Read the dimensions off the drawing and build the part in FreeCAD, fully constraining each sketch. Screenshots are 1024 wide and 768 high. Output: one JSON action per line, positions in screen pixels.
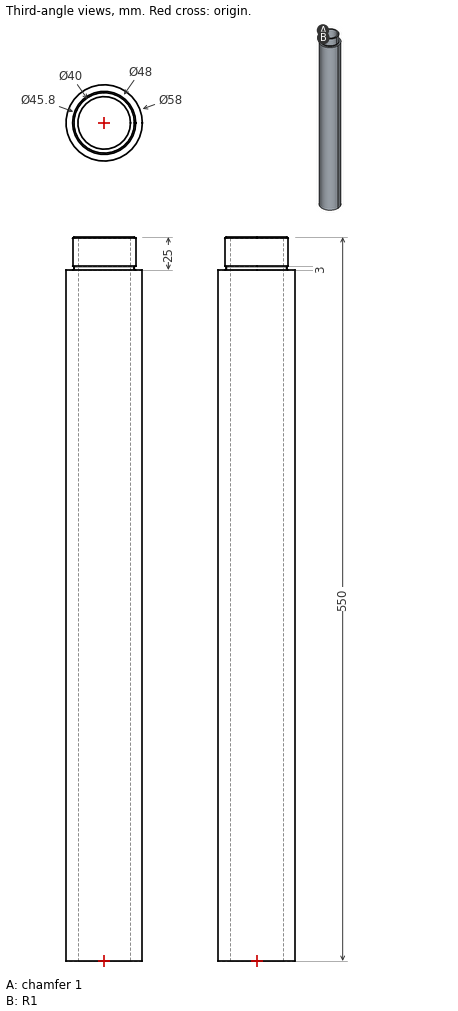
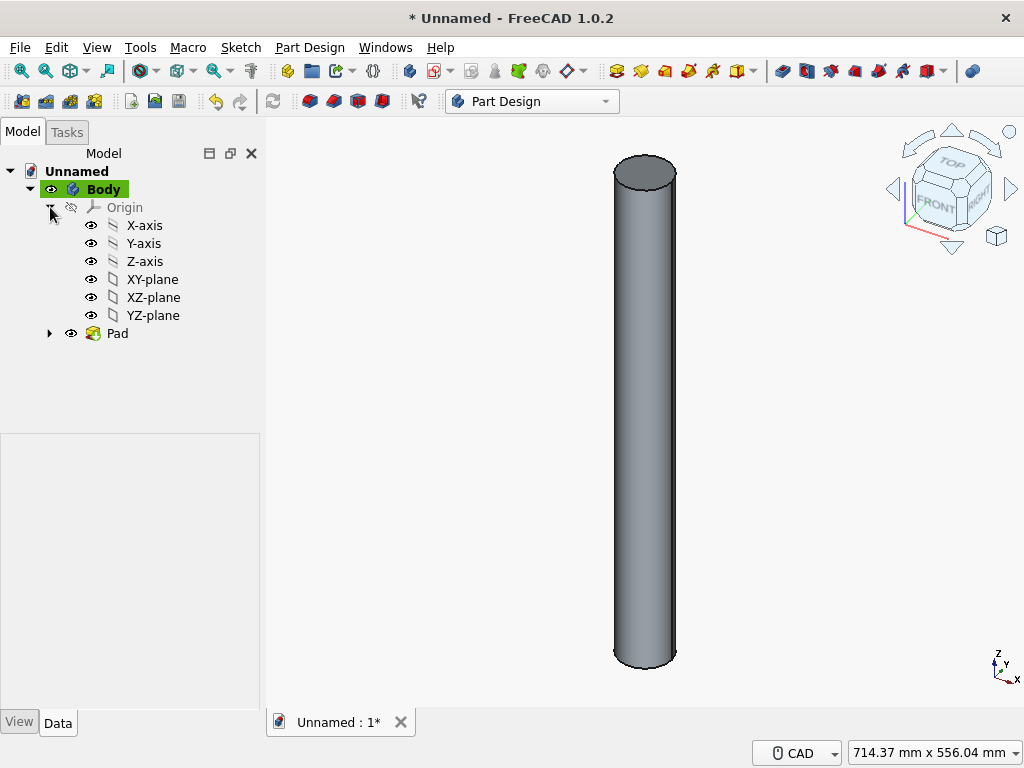
{"action": "left_click", "coordinate": [136, 279]}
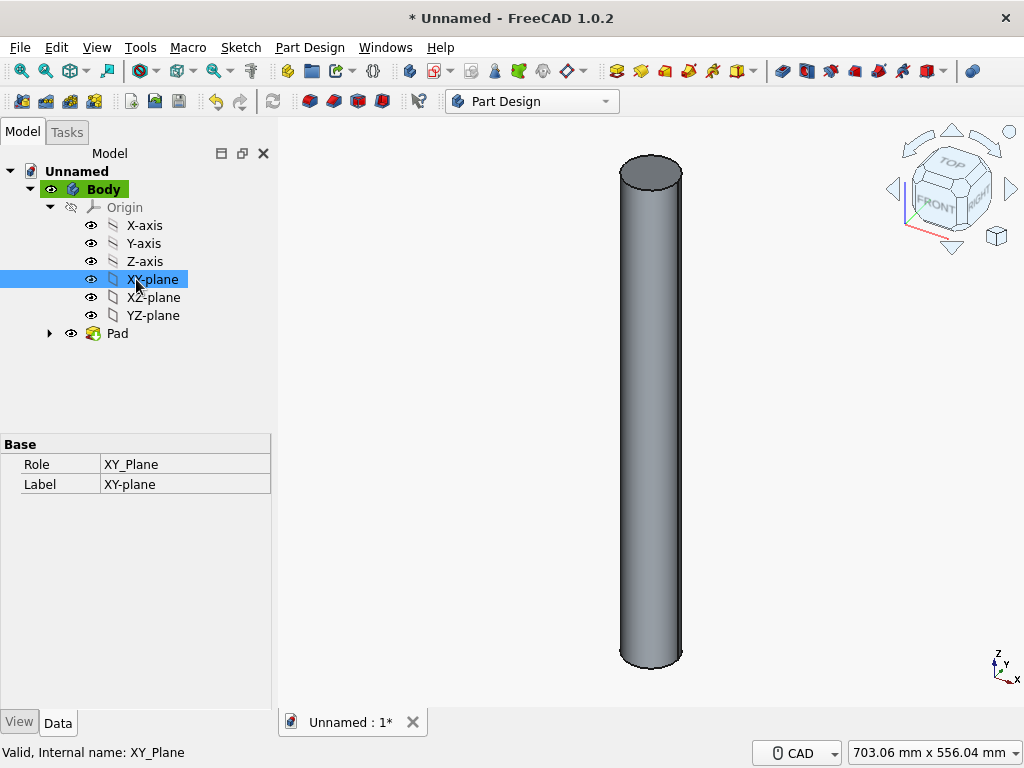
{"action": "left_click", "coordinate": [568, 72]}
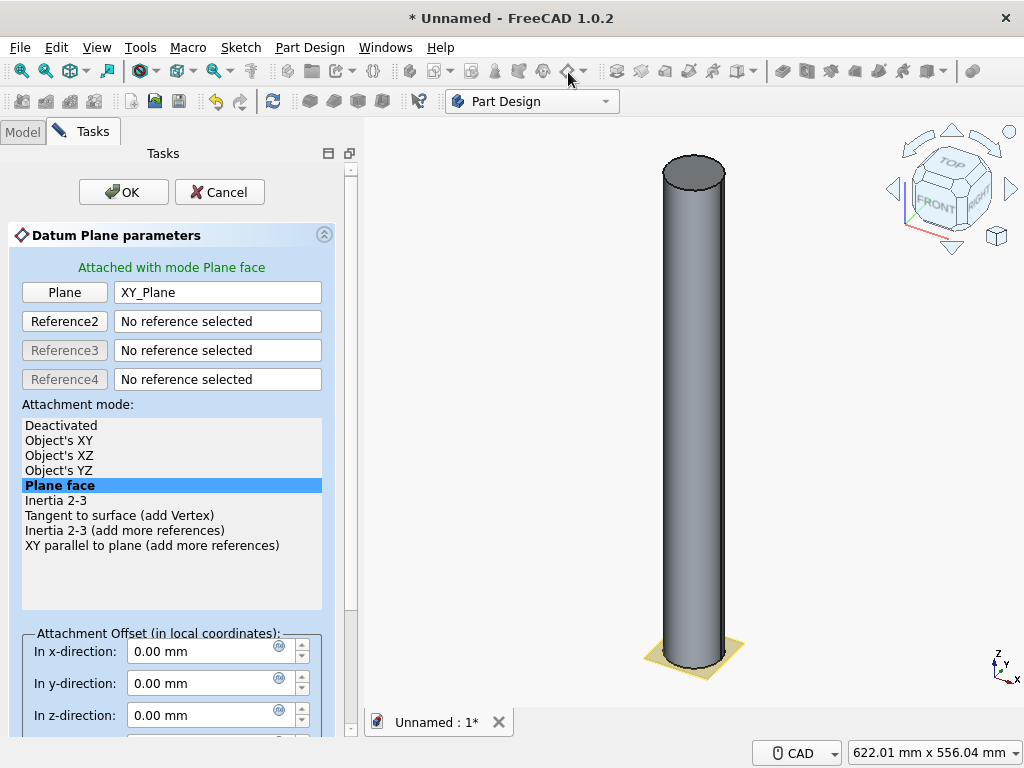
{"action": "triple_click", "coordinate": [210, 715]}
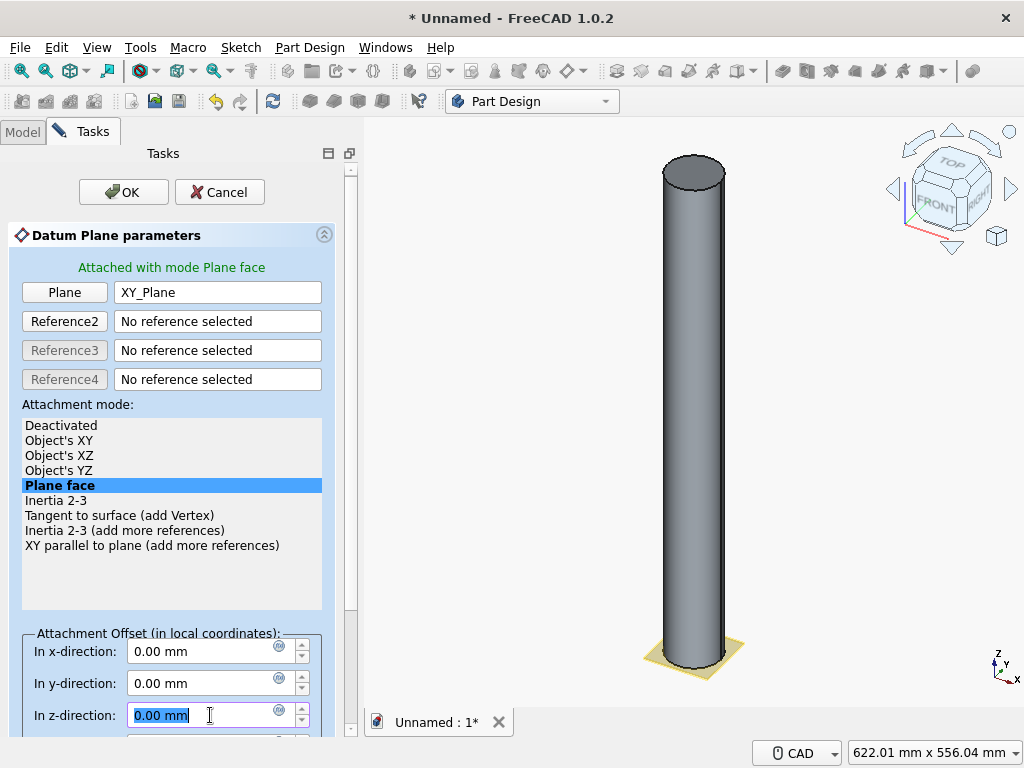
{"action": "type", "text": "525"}
{"action": "key", "text": "Tab"}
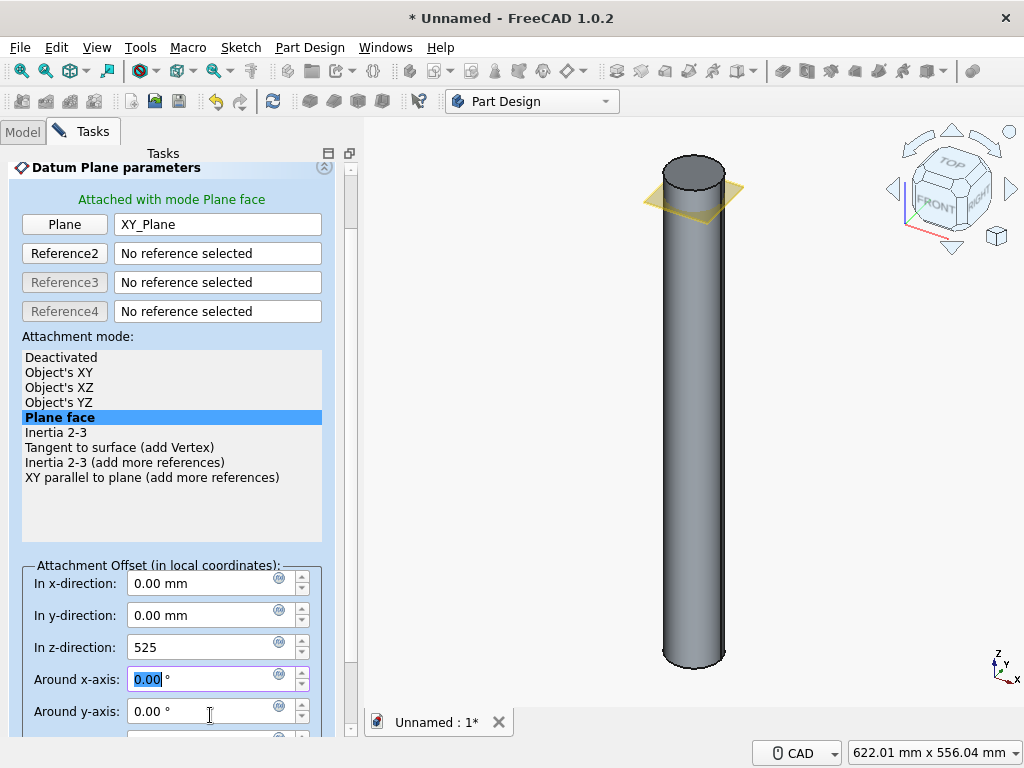
{"action": "scroll", "coordinate": [351, 450], "scroll_direction": "up", "scroll_amount": 2}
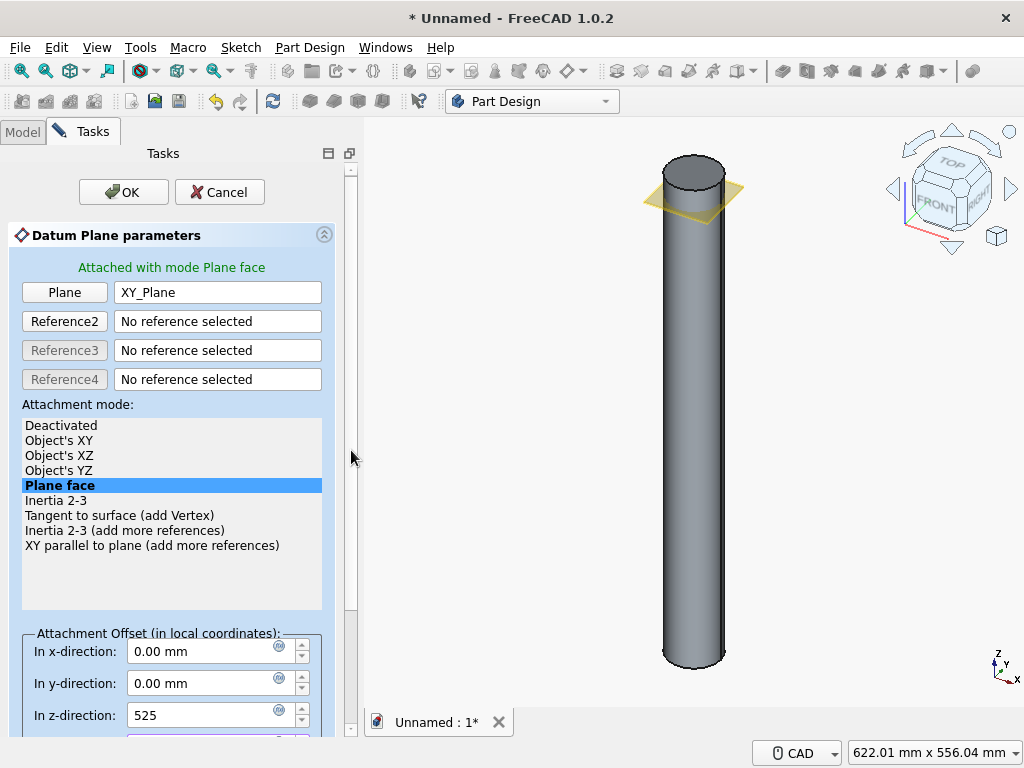
{"action": "left_click", "coordinate": [124, 192]}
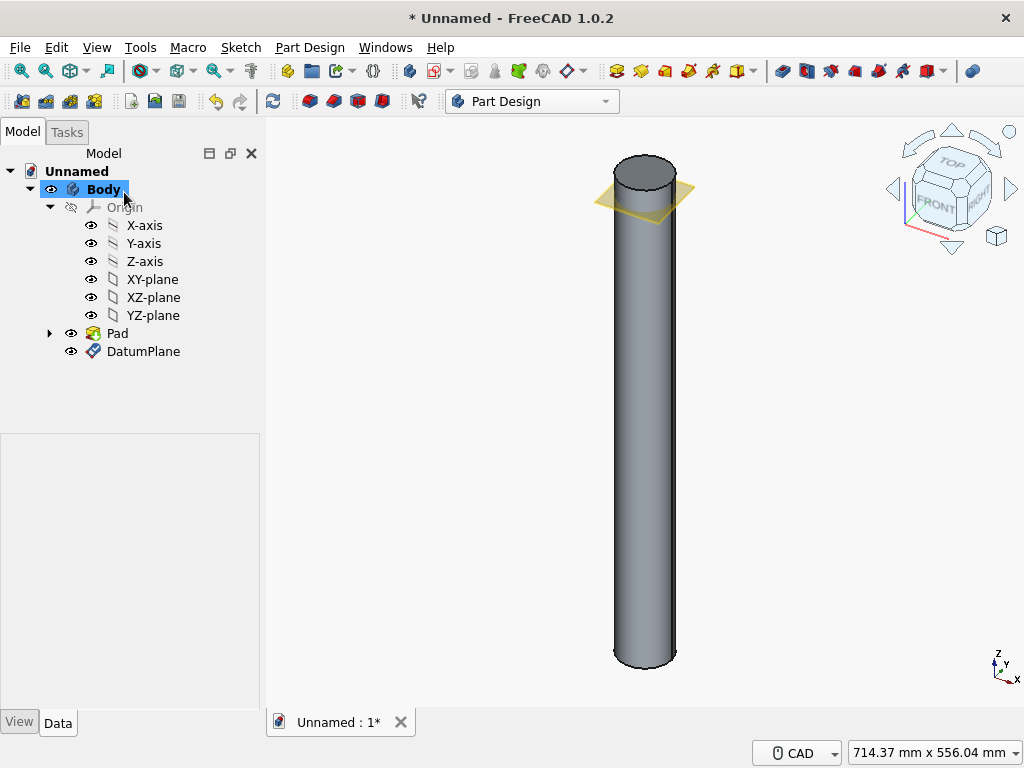
{"action": "left_click", "coordinate": [116, 351]}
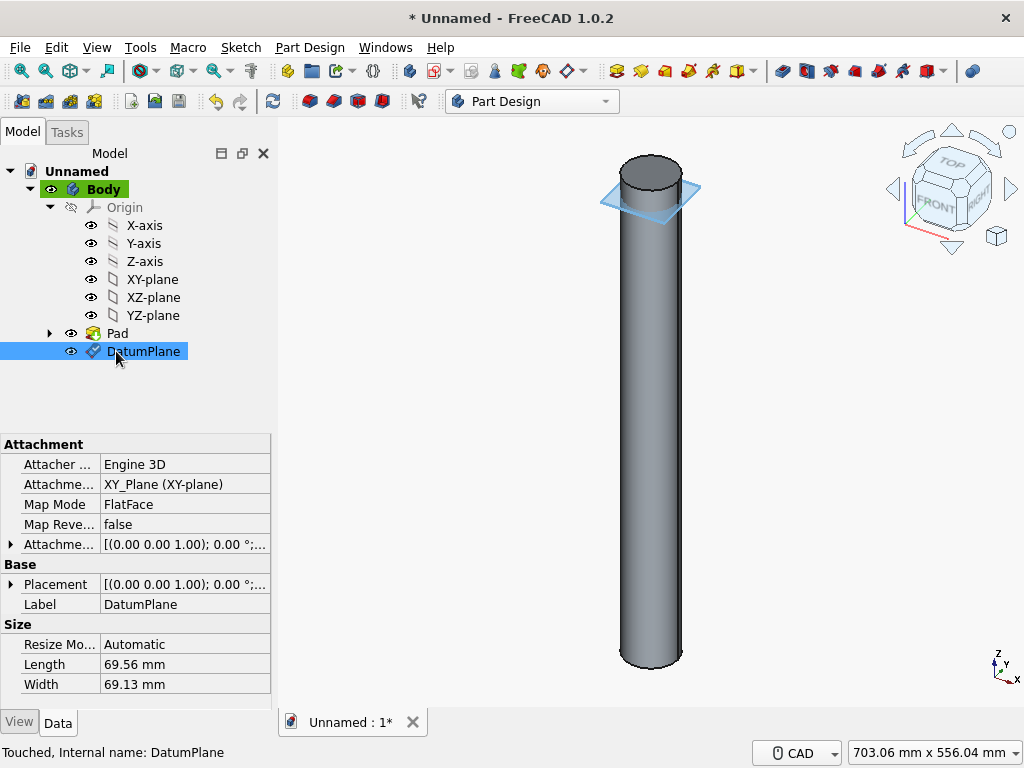
{"action": "left_click", "coordinate": [434, 72]}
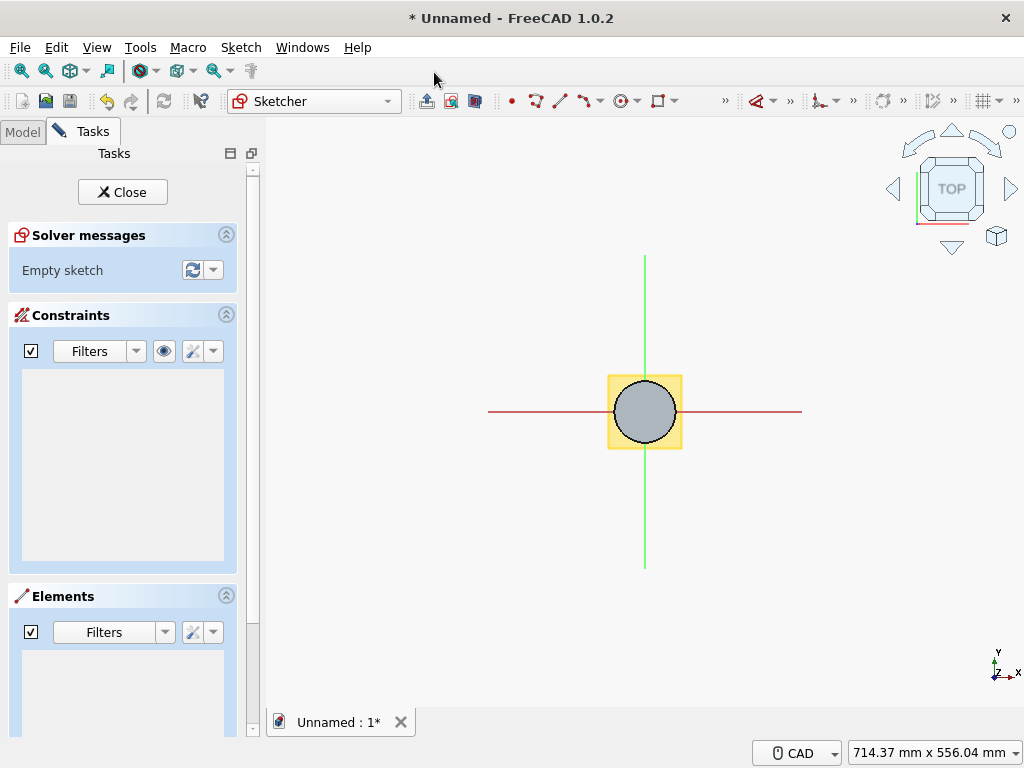
{"action": "left_click", "coordinate": [476, 102]}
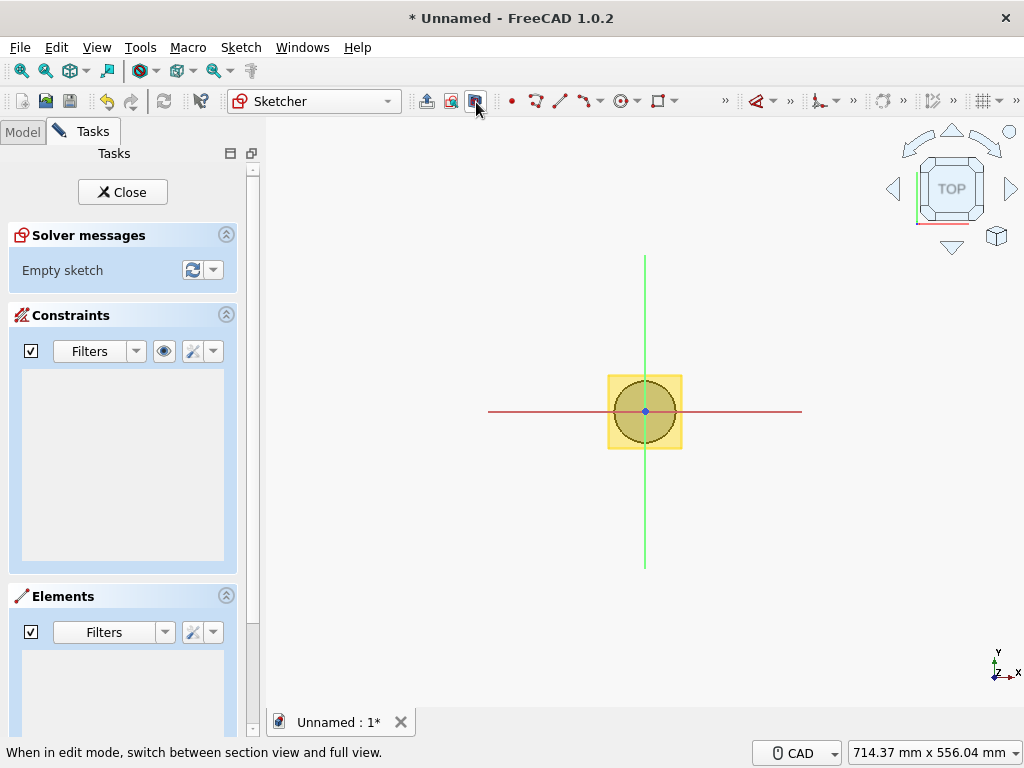
{"action": "scroll", "coordinate": [659, 412], "scroll_direction": "up", "scroll_amount": 9}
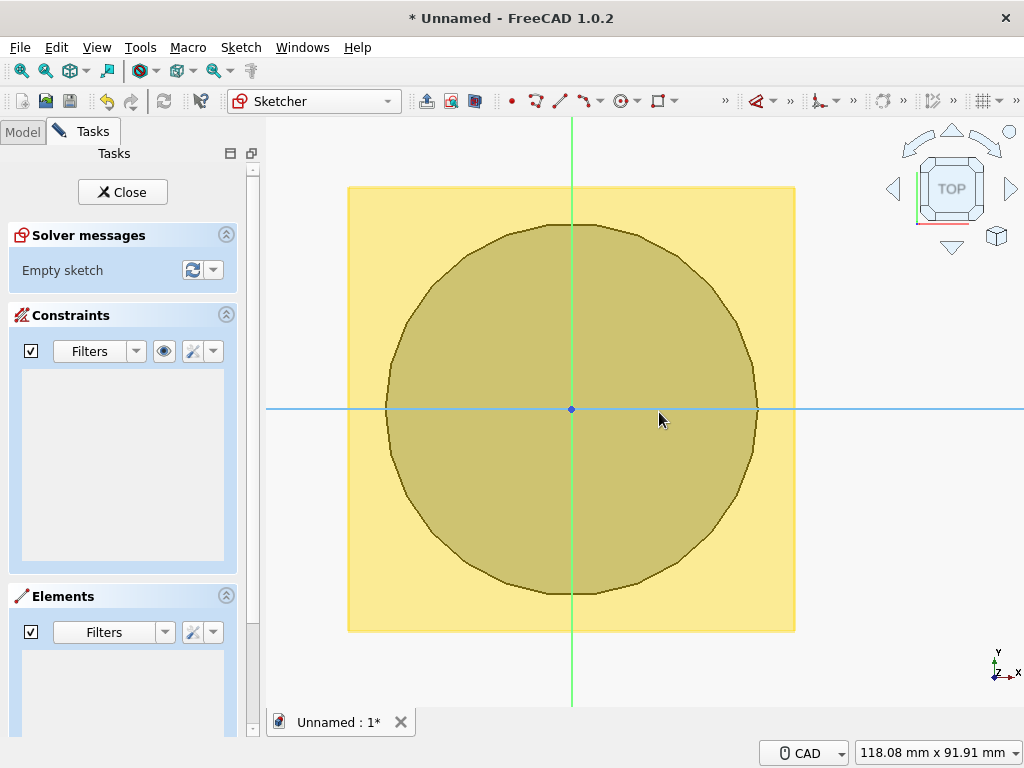
{"action": "left_click", "coordinate": [622, 102]}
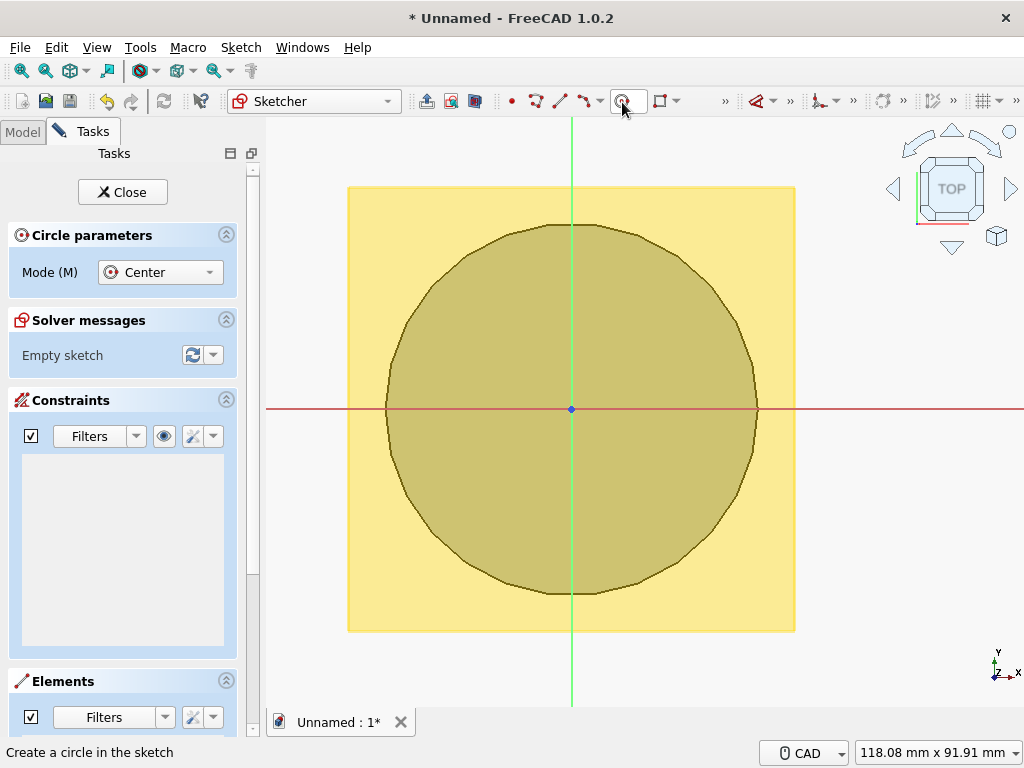
{"action": "left_click", "coordinate": [572, 409]}
{"action": "mouse_move", "coordinate": [703, 278]}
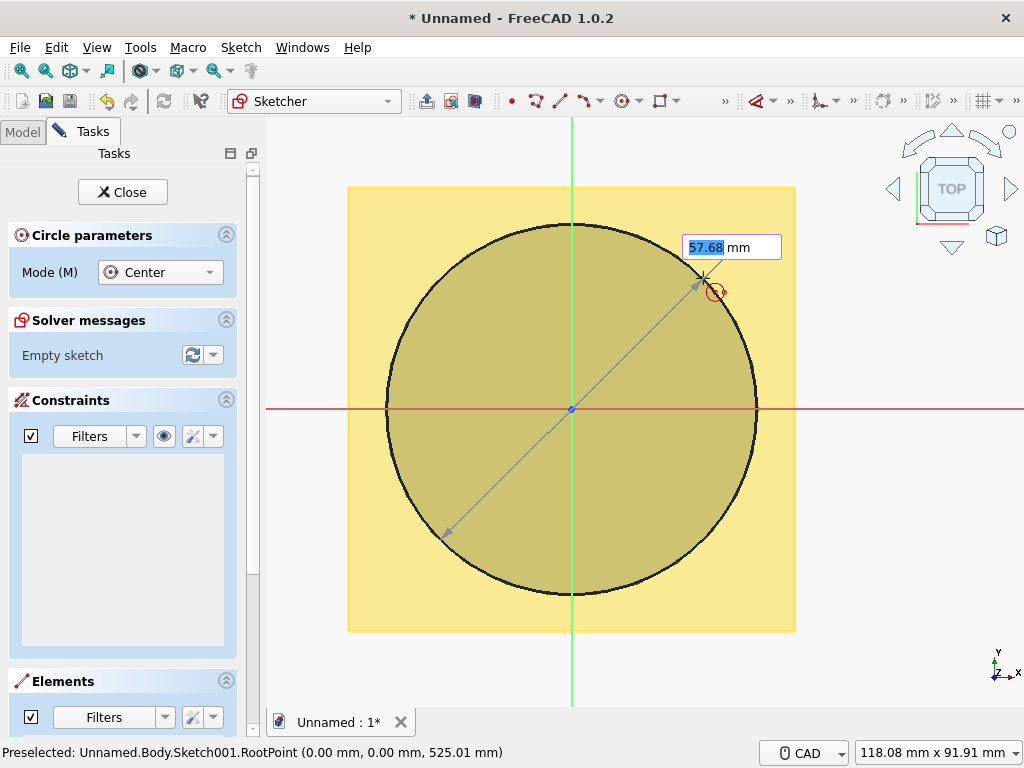
{"action": "type", "text": "58"}
{"action": "key", "text": "Return"}